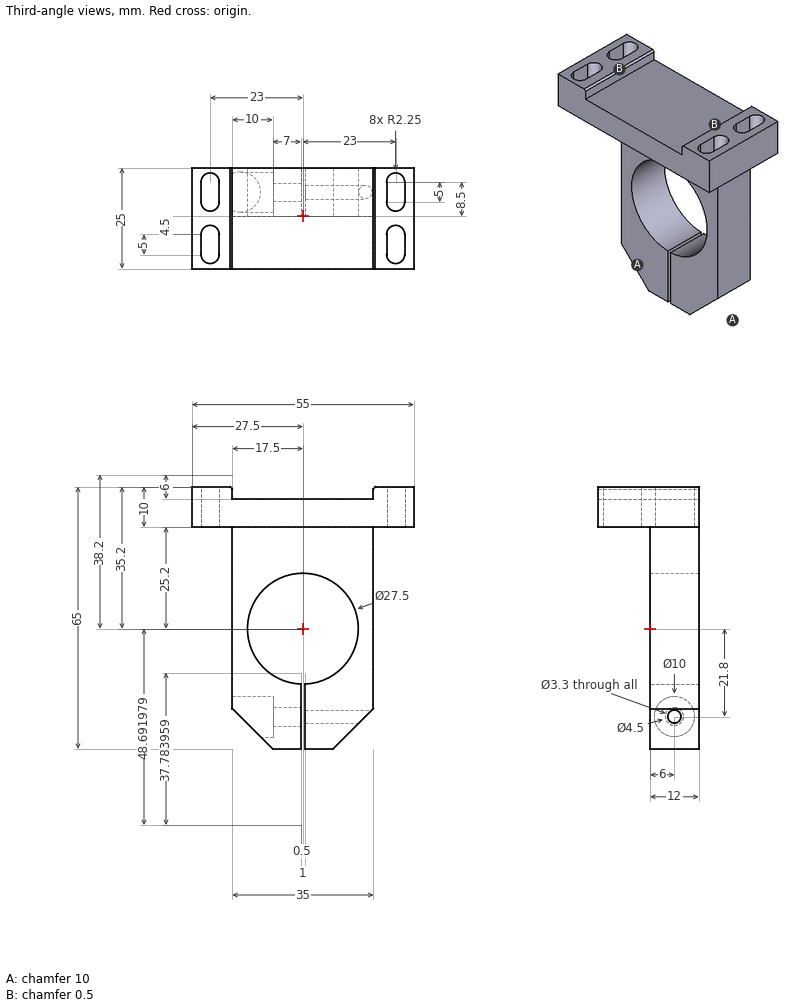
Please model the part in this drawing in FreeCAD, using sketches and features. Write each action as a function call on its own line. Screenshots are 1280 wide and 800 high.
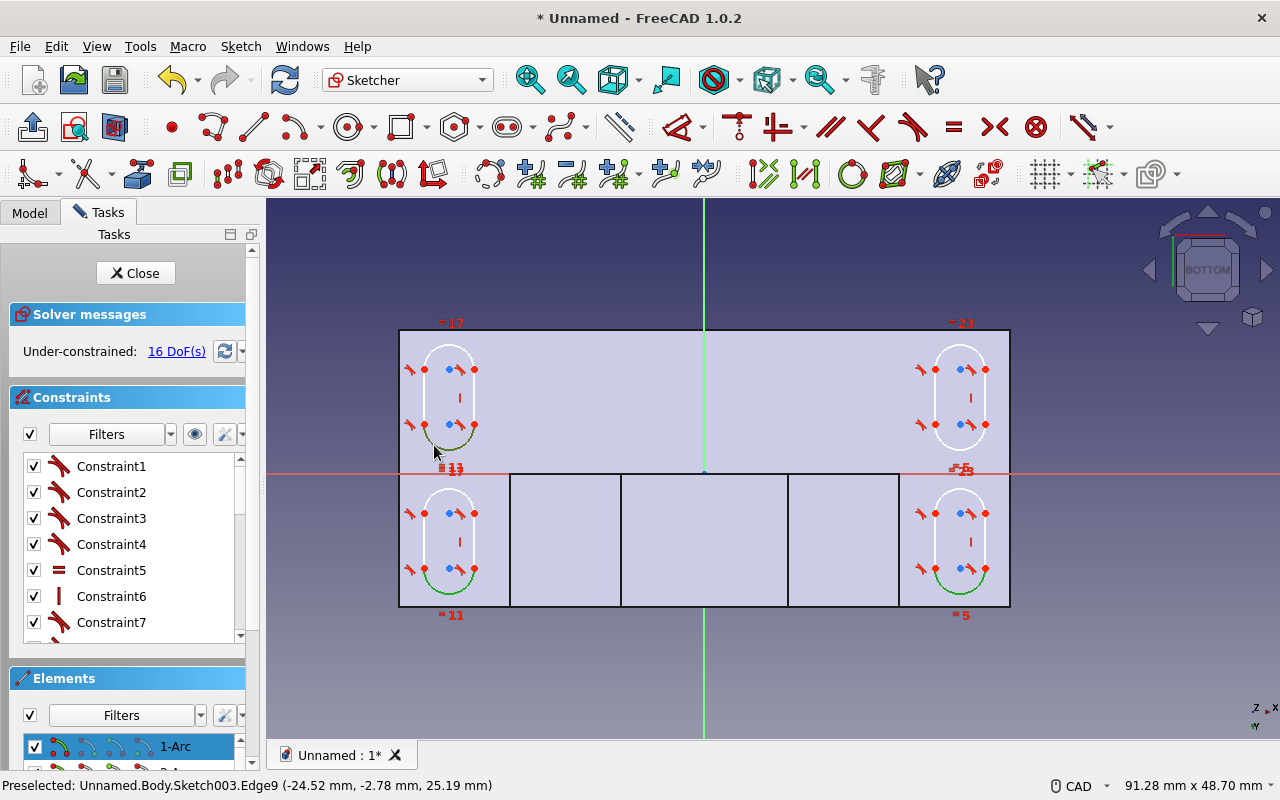
click(945, 445)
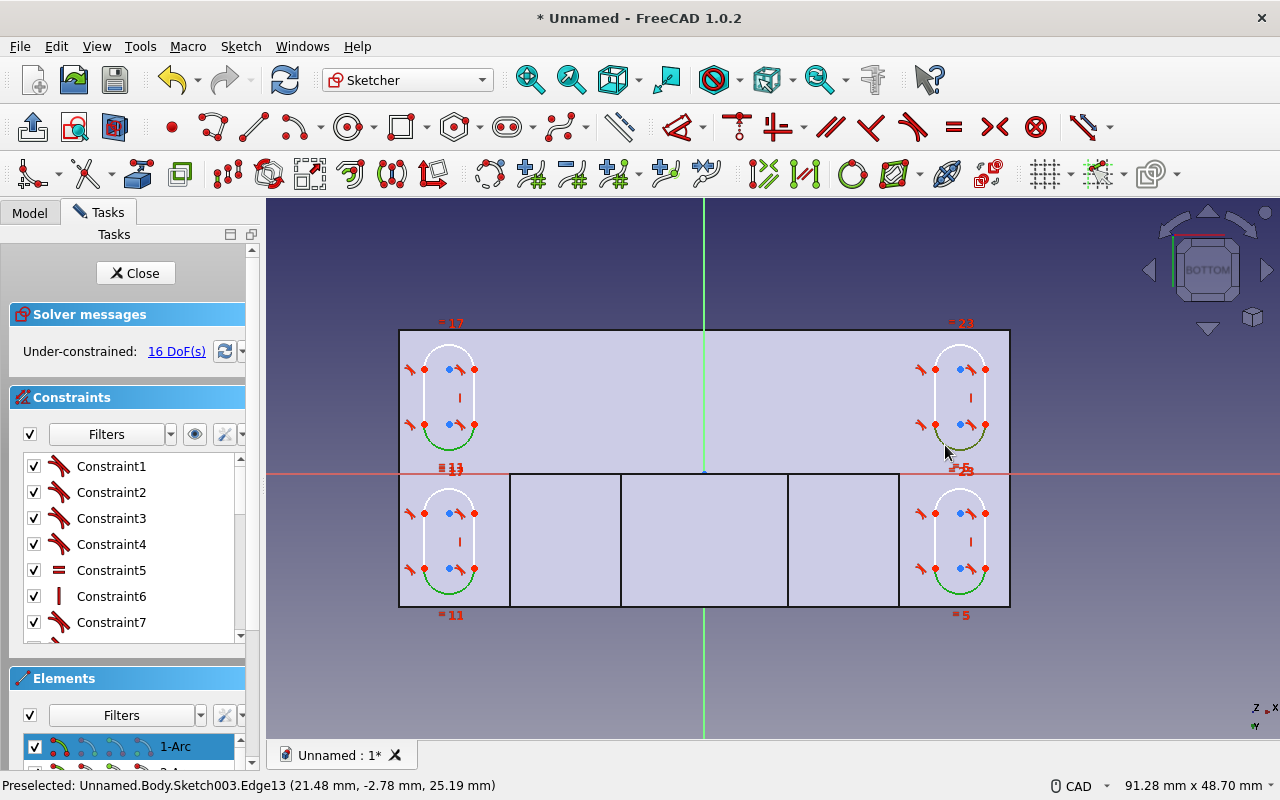
click(954, 128)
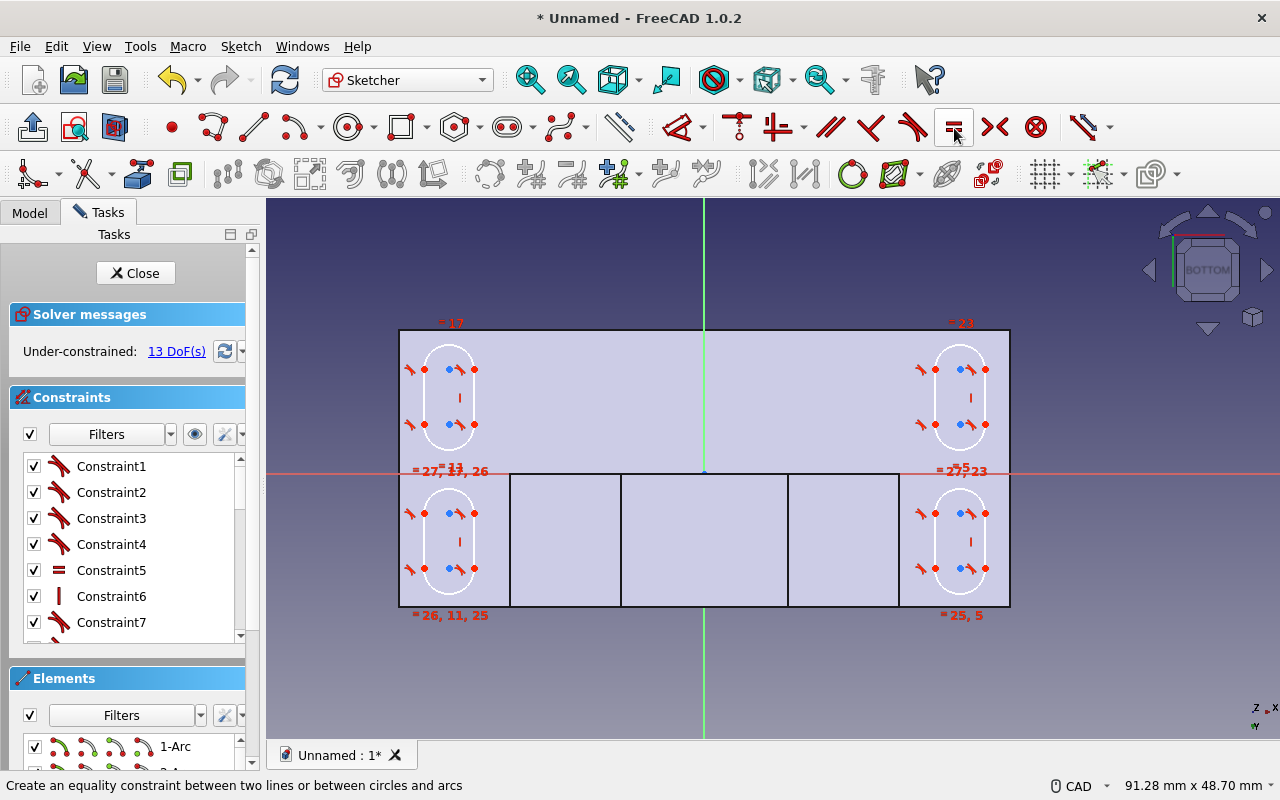
click(676, 128)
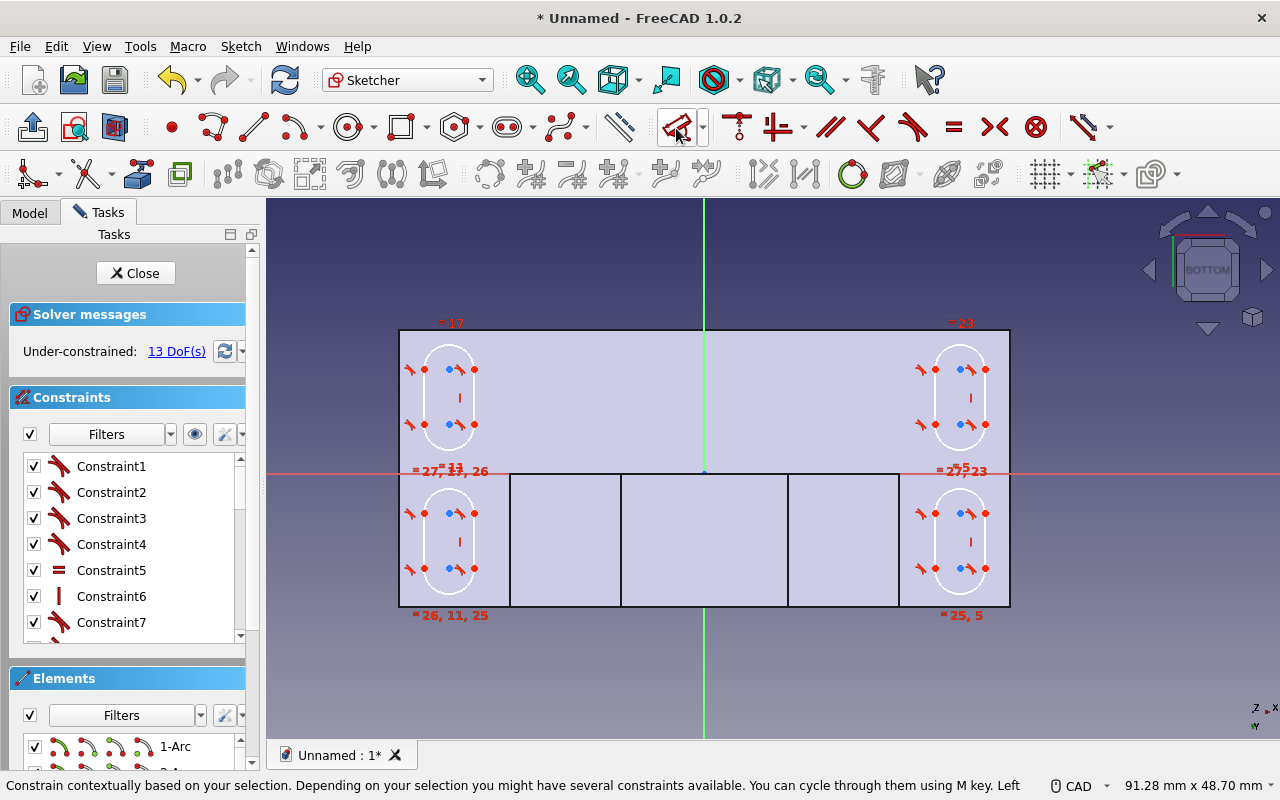
scroll(945, 589, up, 3)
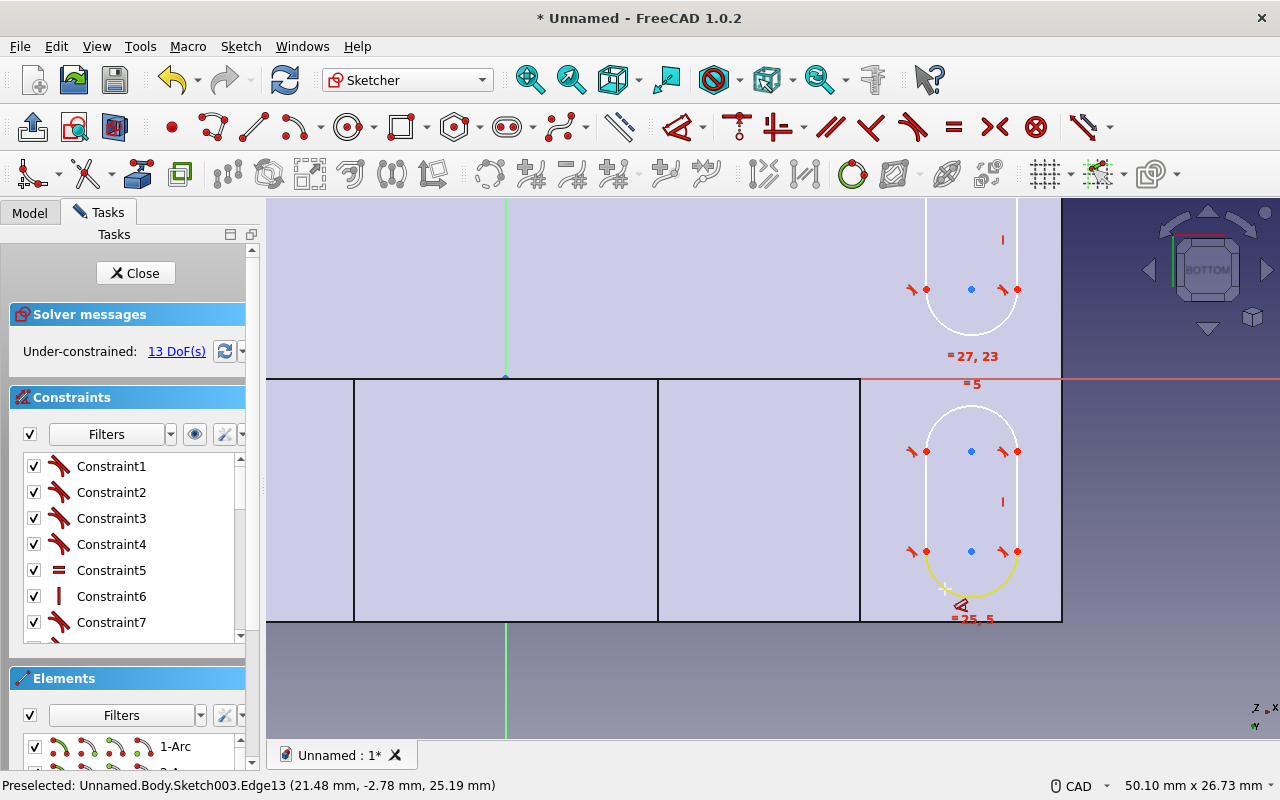
click(945, 589)
click(926, 615)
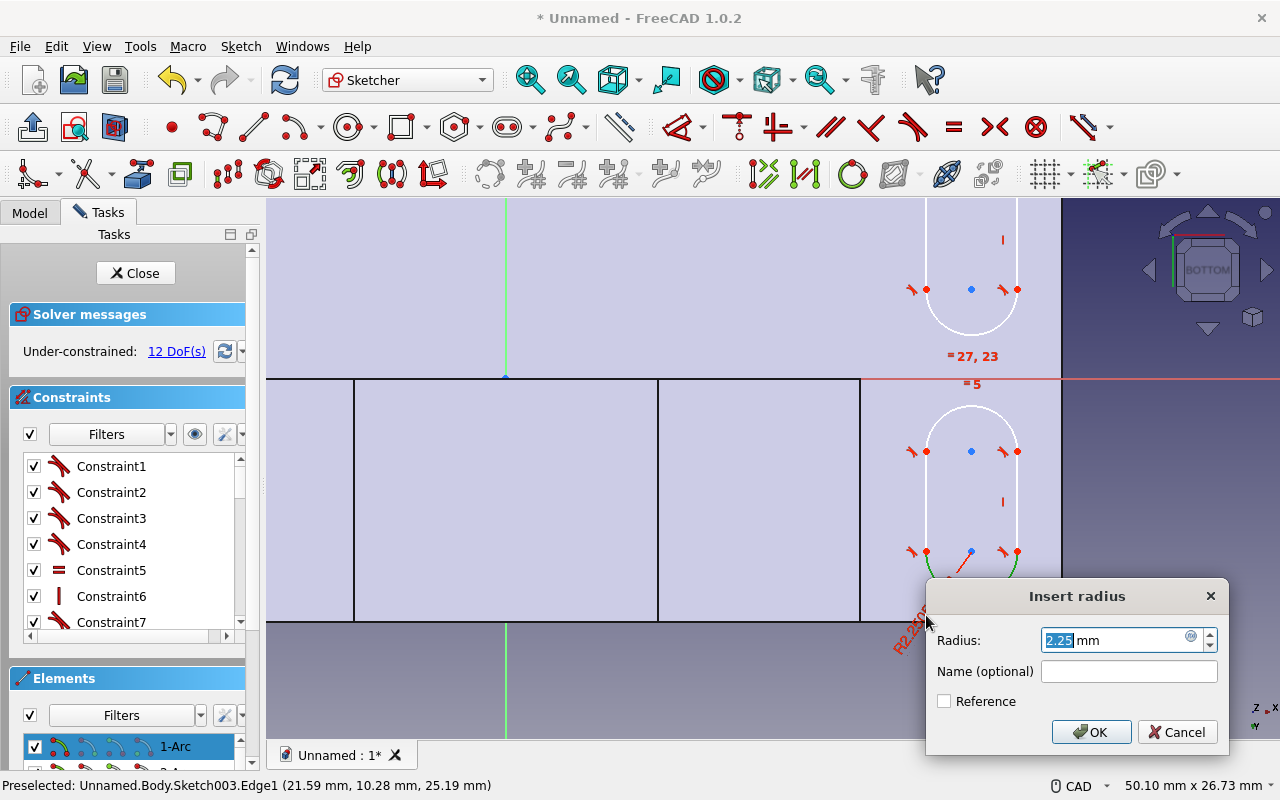
text(2.25)
key(Return)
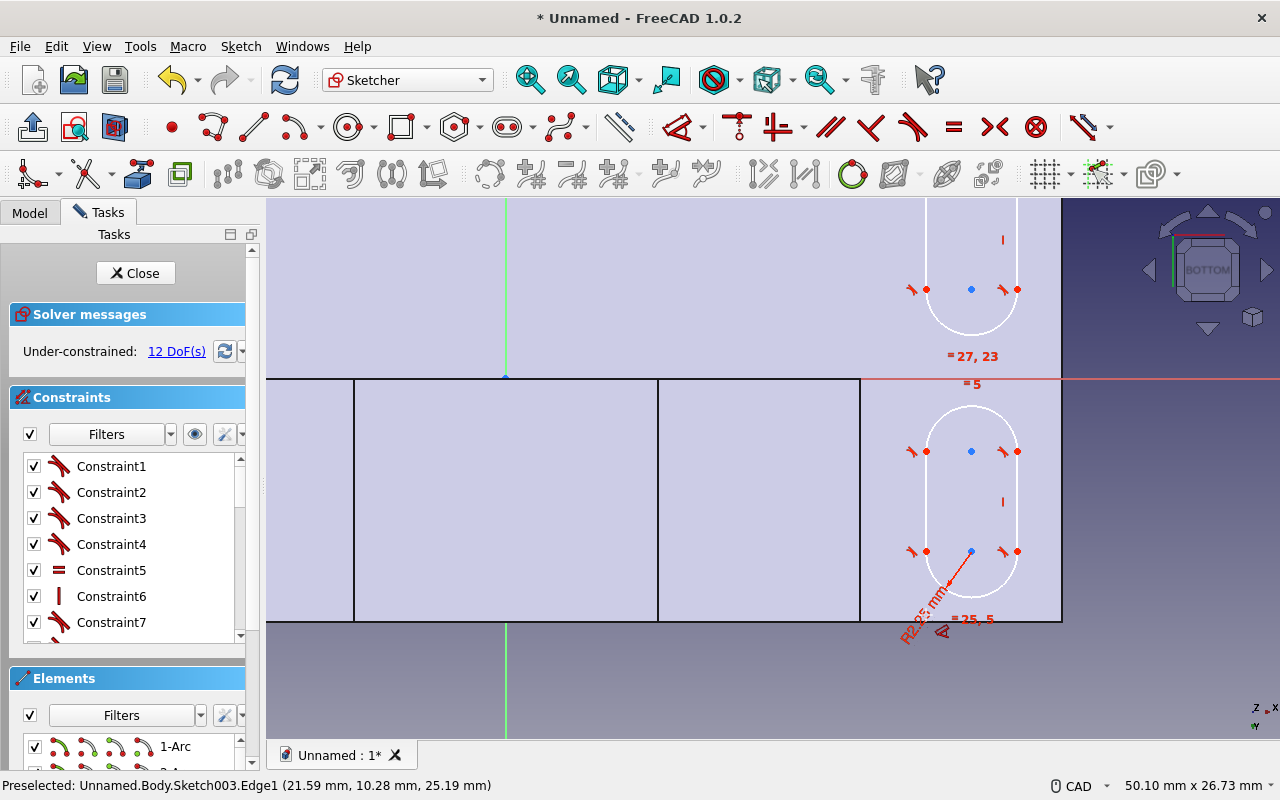
click(926, 522)
click(960, 502)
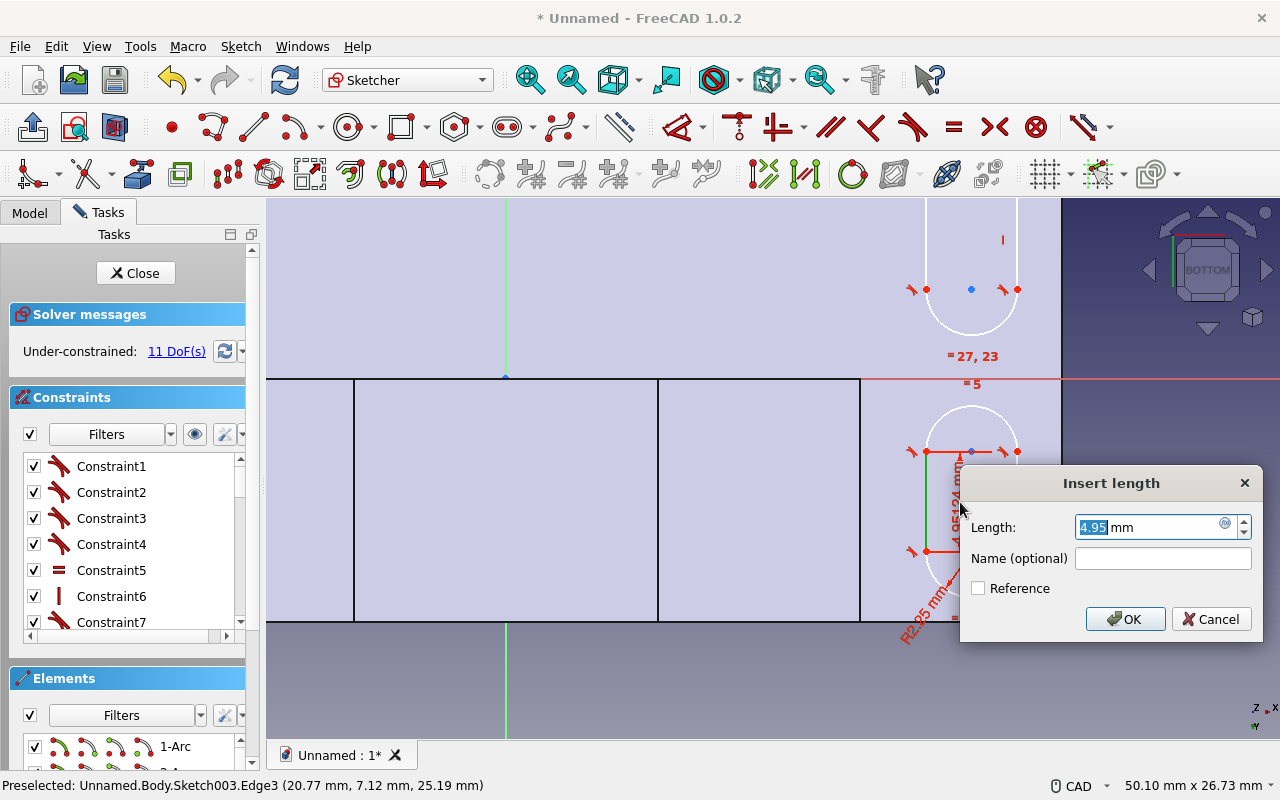
text(5)
key(Return)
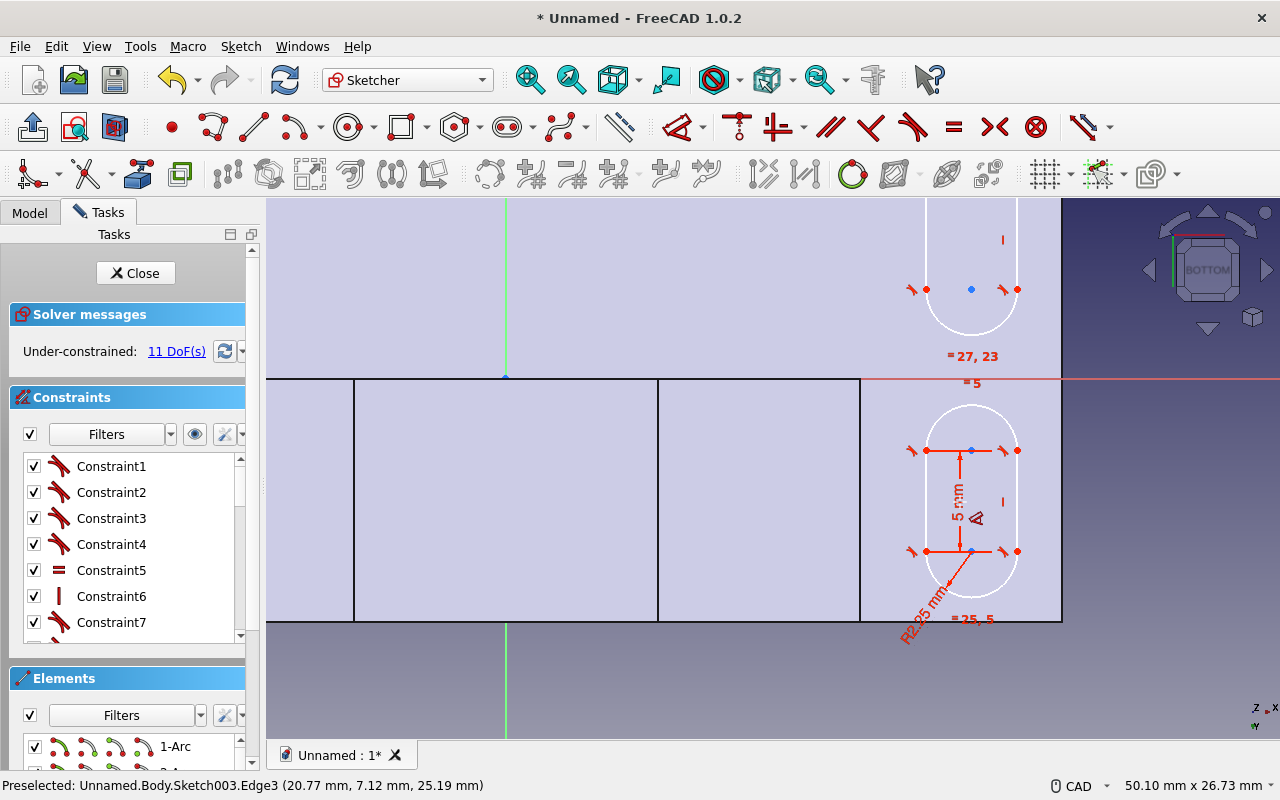
scroll(946, 590, down, 3)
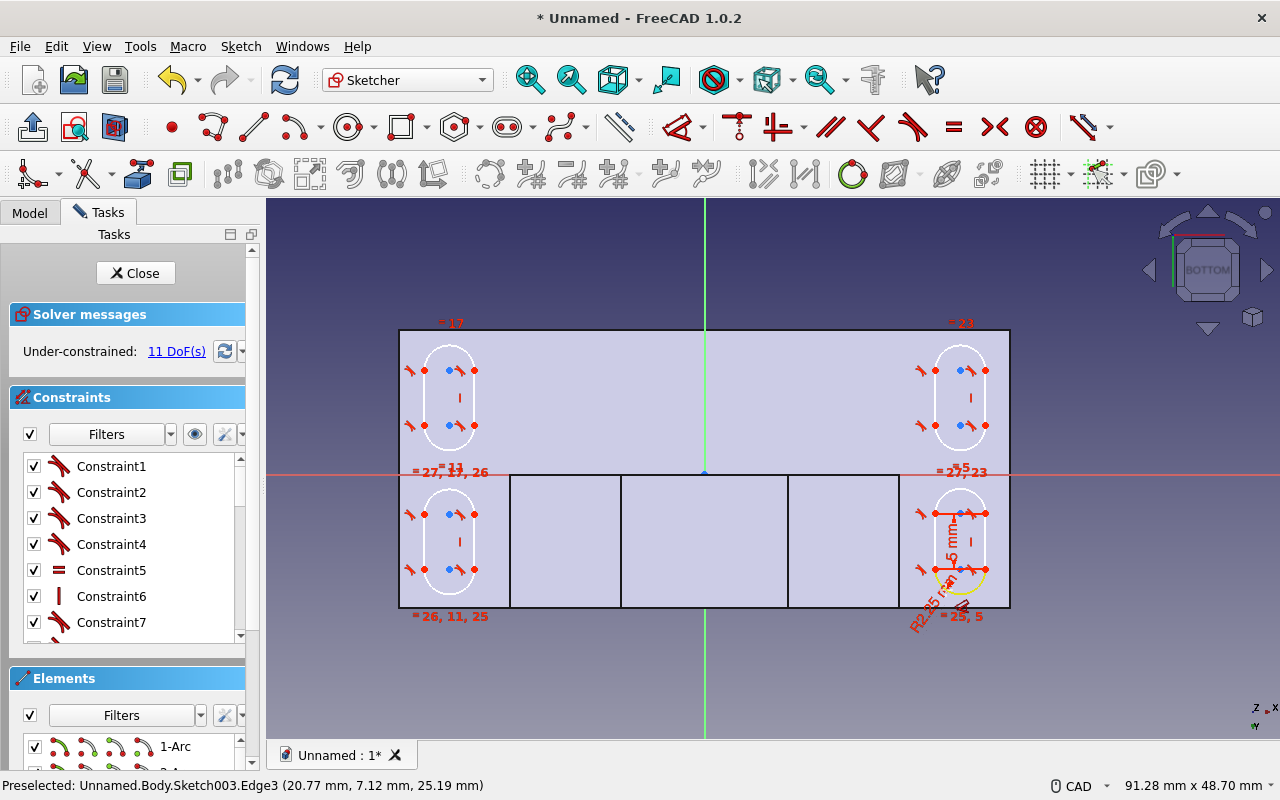
click(424, 553)
click(390, 542)